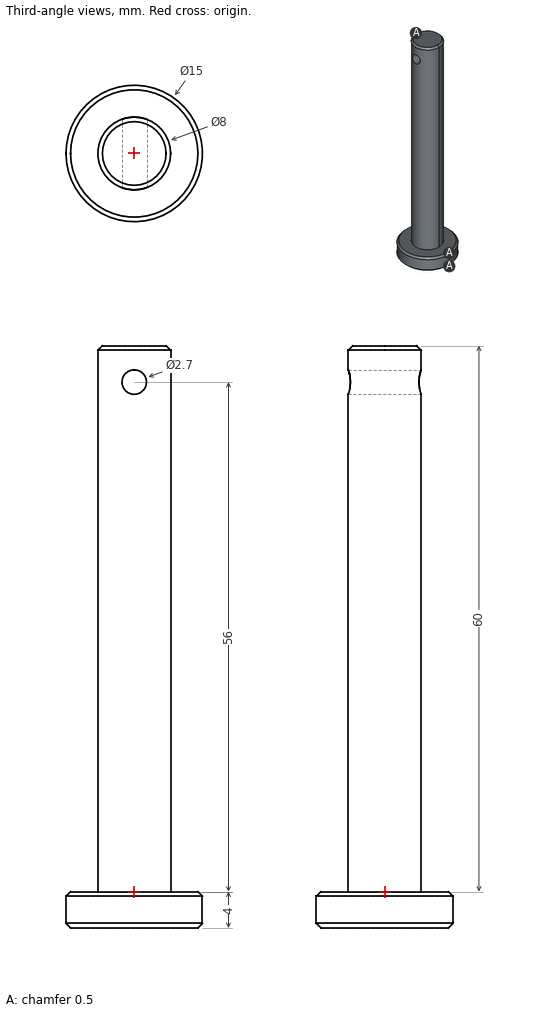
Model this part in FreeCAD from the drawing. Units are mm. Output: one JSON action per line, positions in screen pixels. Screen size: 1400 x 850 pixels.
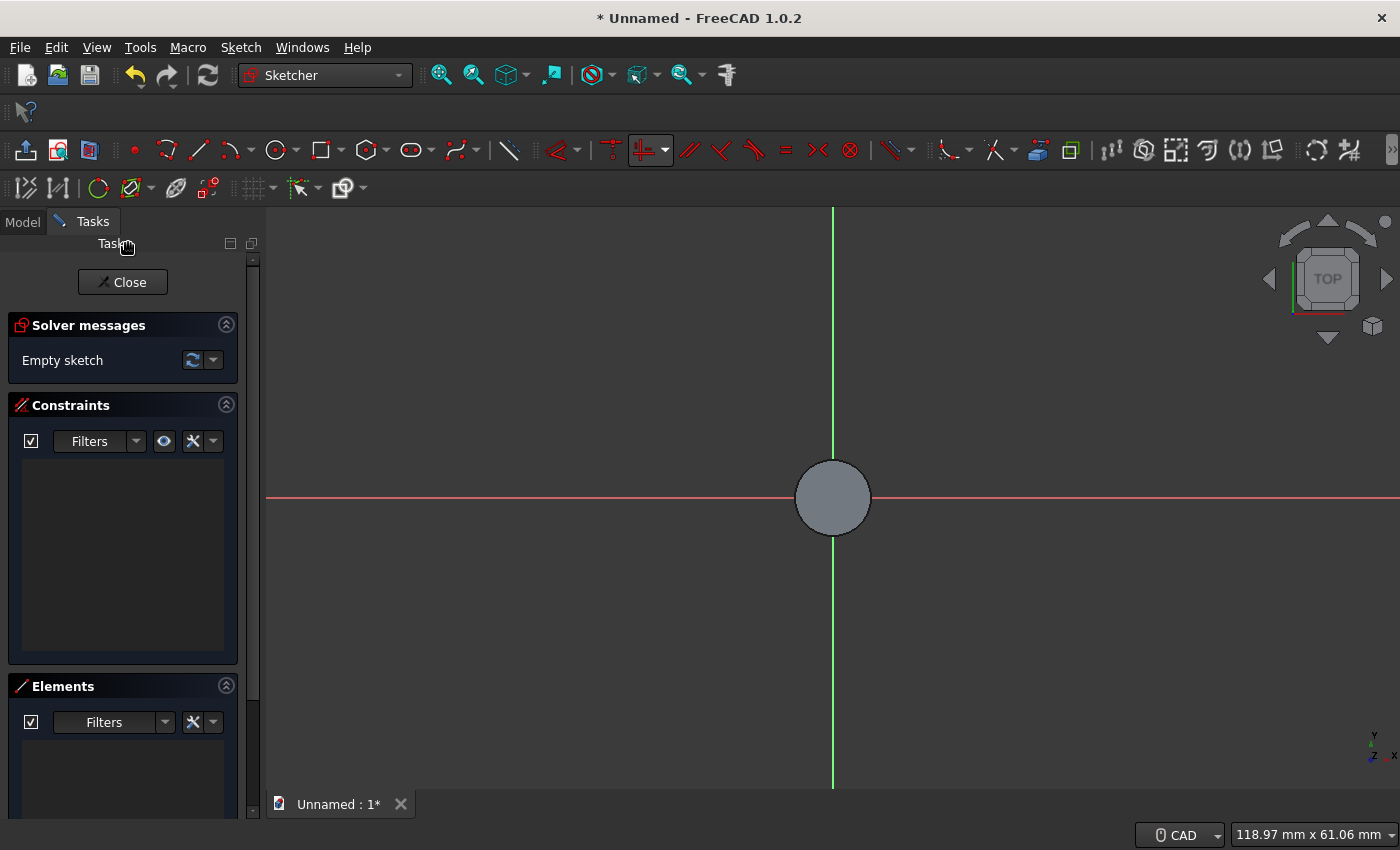
{"action": "left_click", "coordinate": [90, 150]}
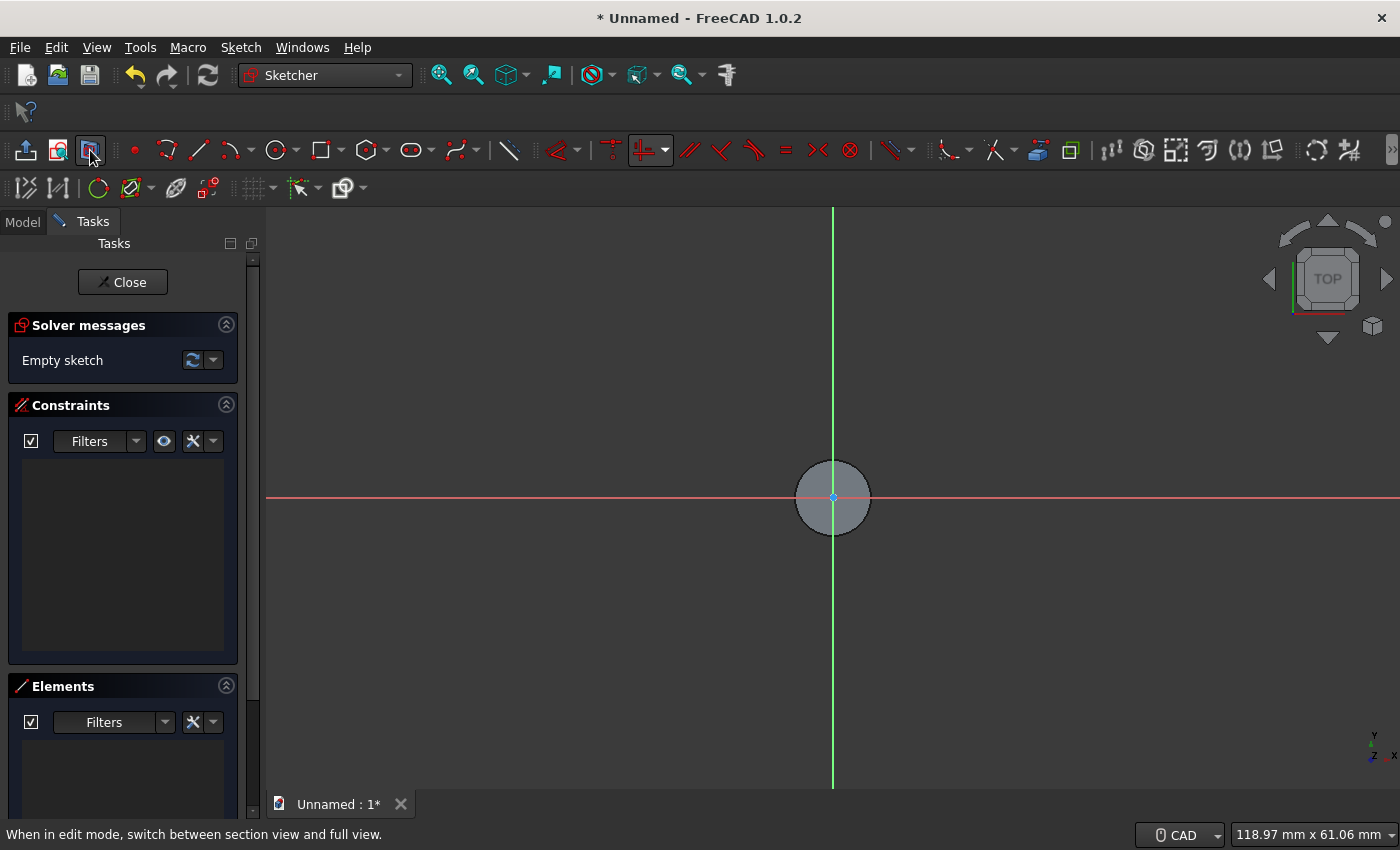
{"action": "scroll", "coordinate": [873, 498], "scroll_direction": "up", "scroll_amount": 5}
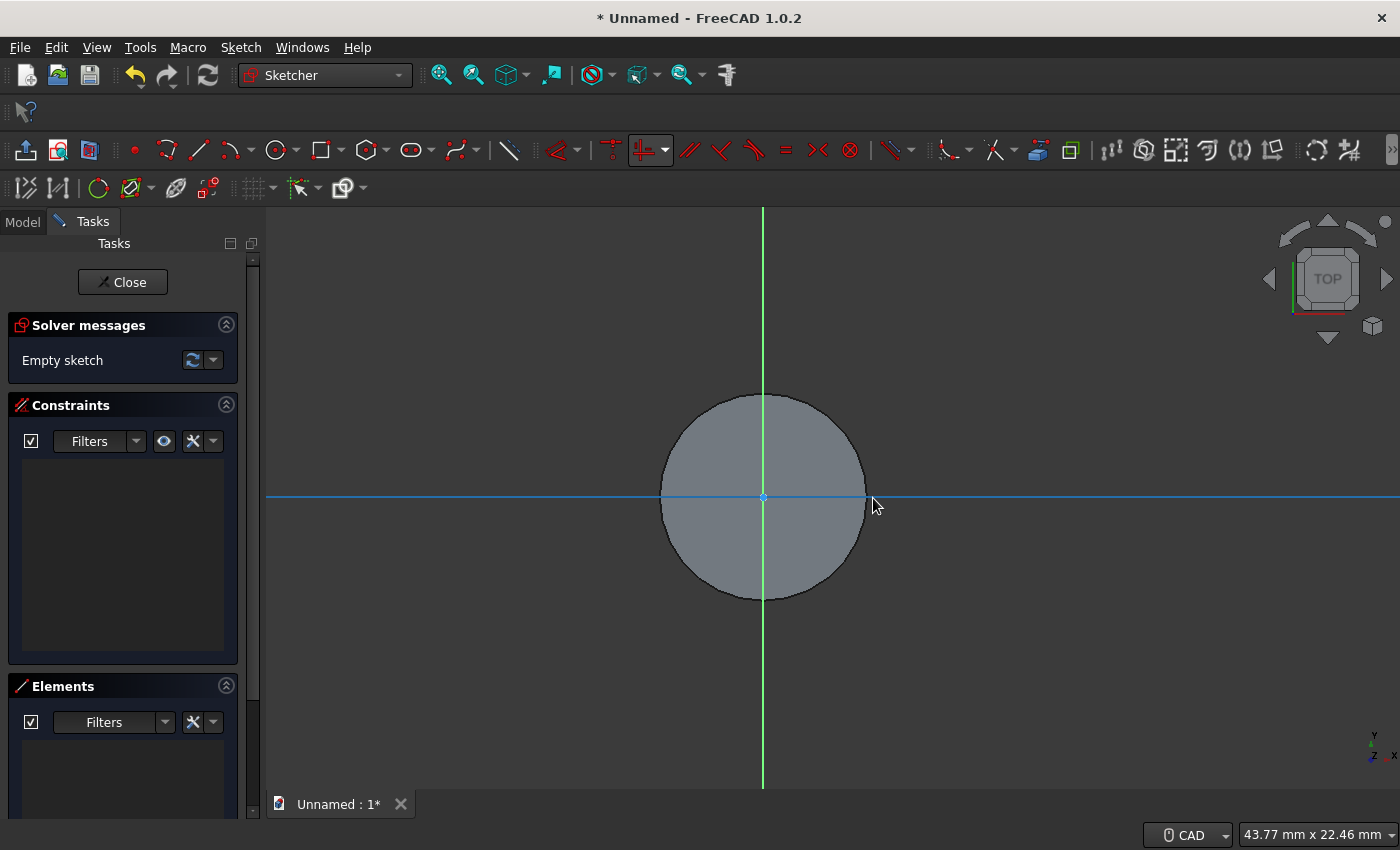
{"action": "left_click", "coordinate": [276, 150]}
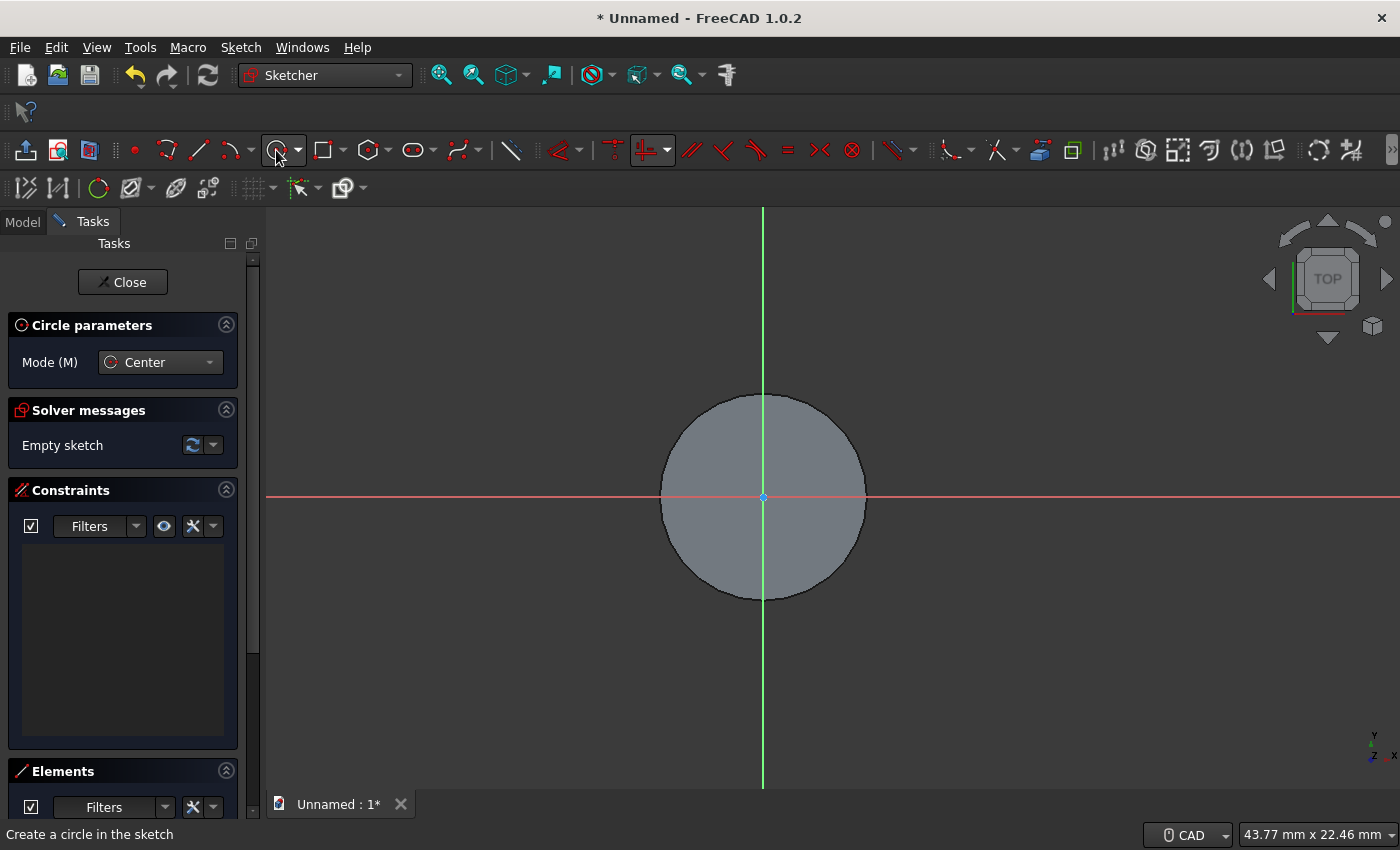
{"action": "left_click", "coordinate": [763, 497]}
{"action": "left_click", "coordinate": [901, 360]}
{"action": "key", "text": "Escape"}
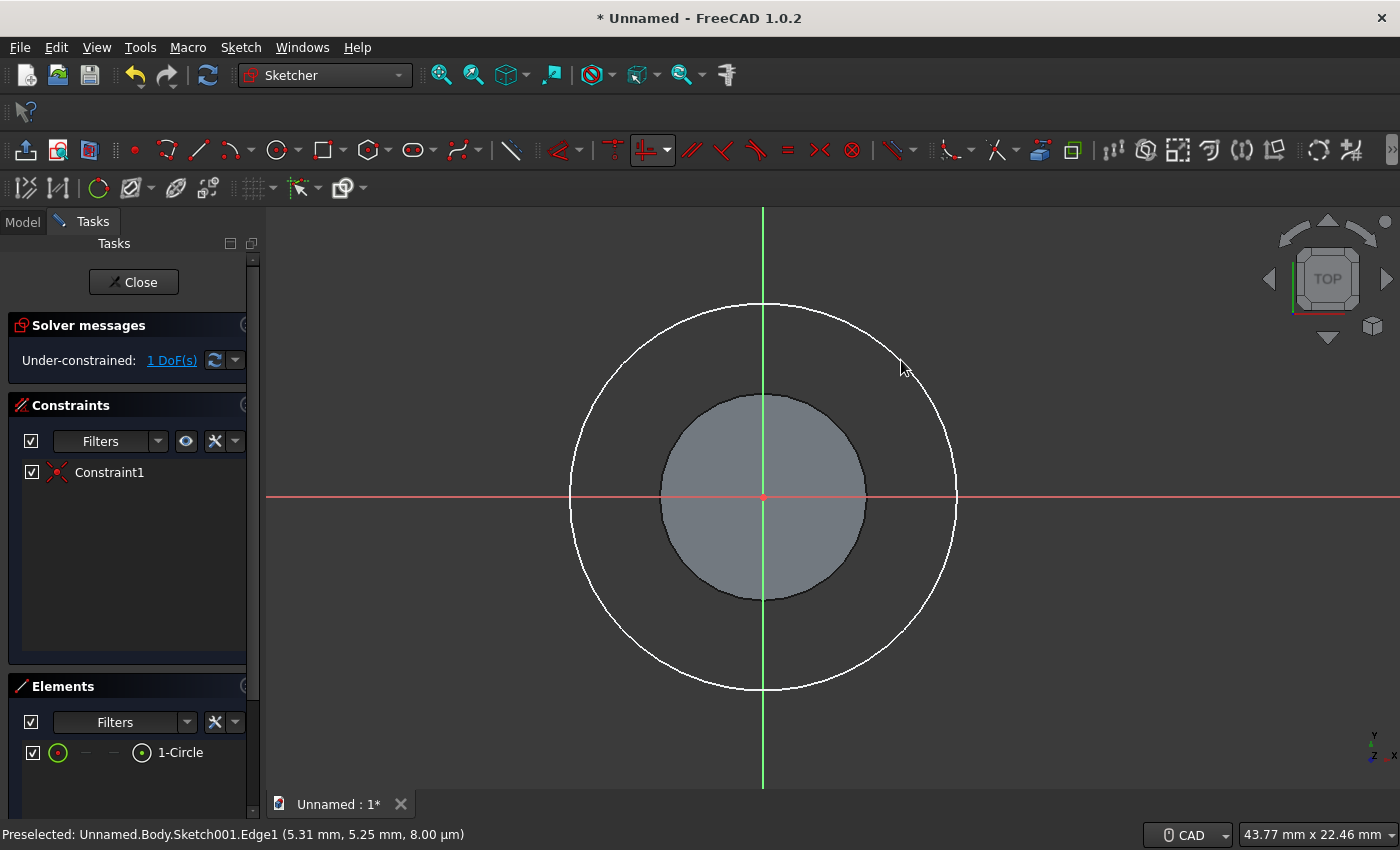
{"action": "left_click", "coordinate": [558, 150]}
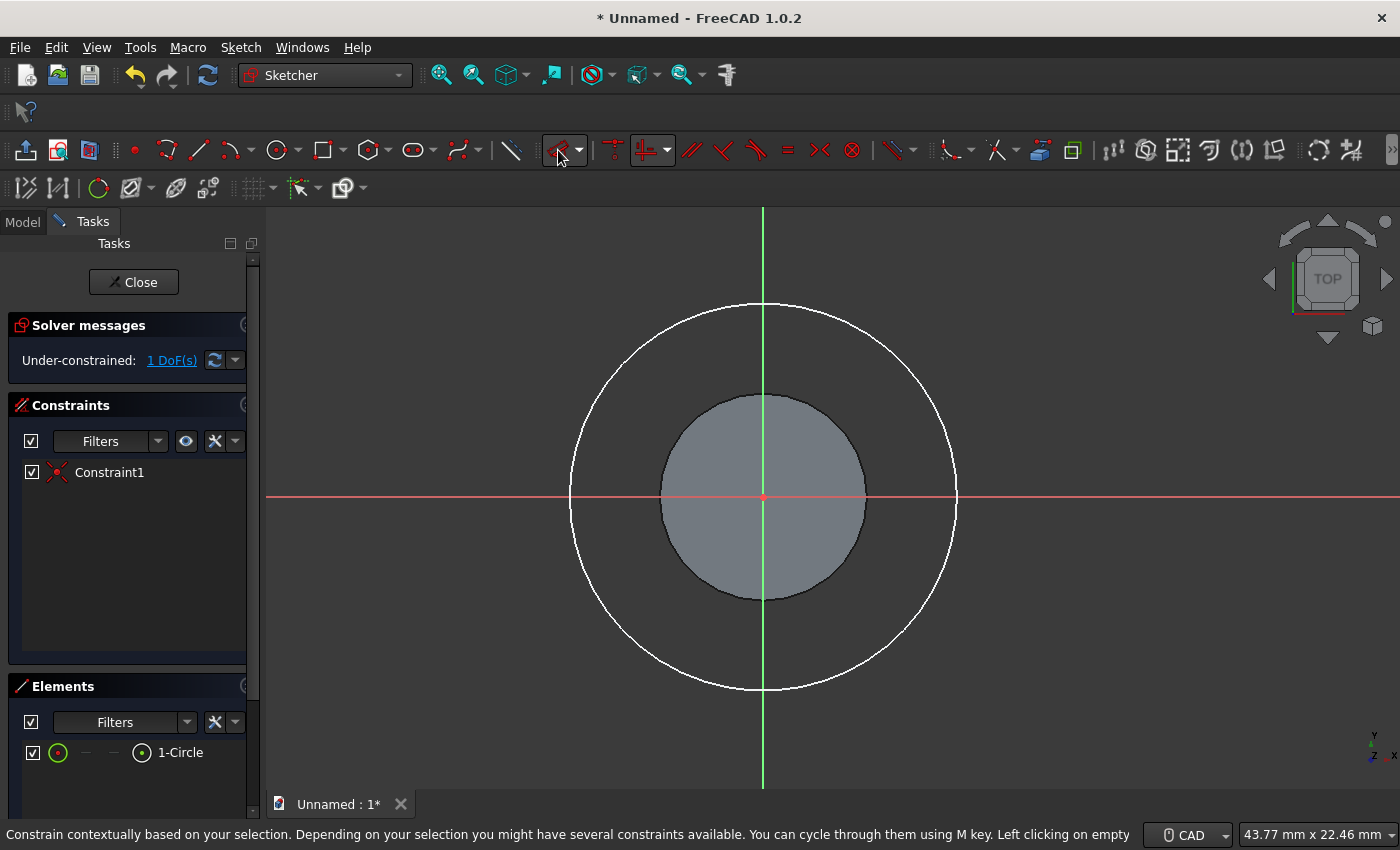
{"action": "left_click", "coordinate": [900, 360]}
{"action": "left_click", "coordinate": [923, 337]}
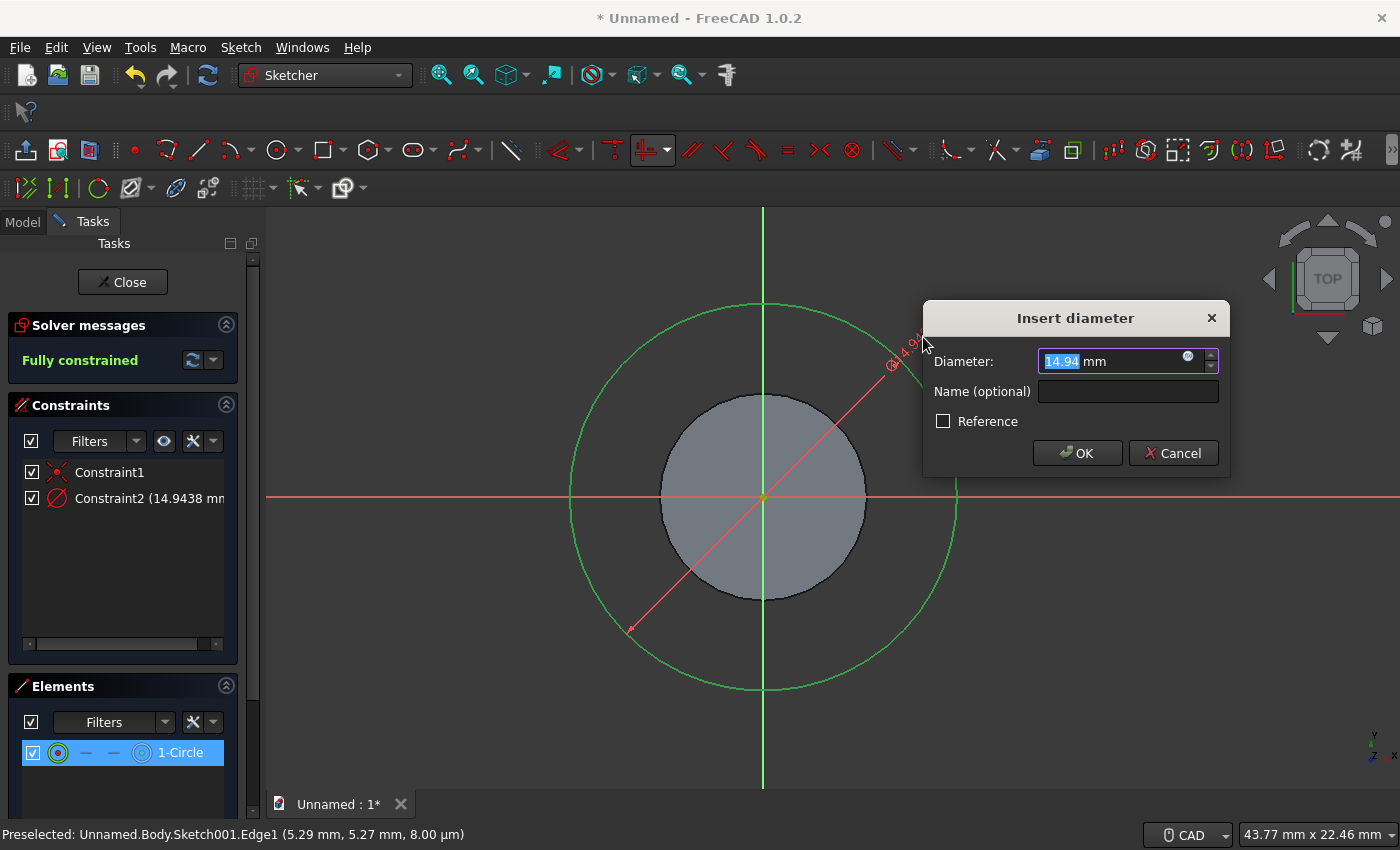
{"action": "type", "text": "15"}
{"action": "key", "text": "Return"}
{"action": "key", "text": "Escape"}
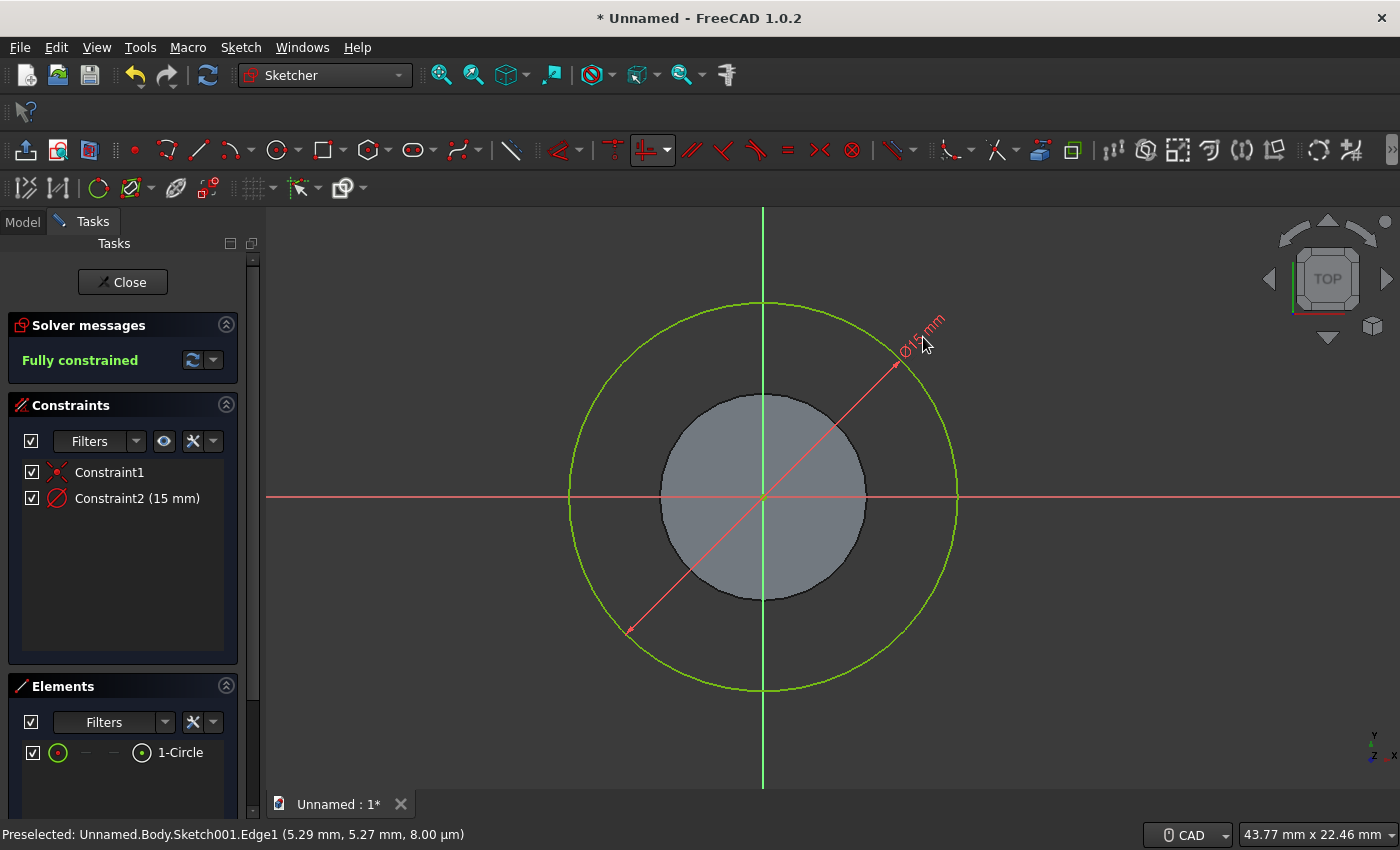
{"action": "left_click", "coordinate": [123, 282]}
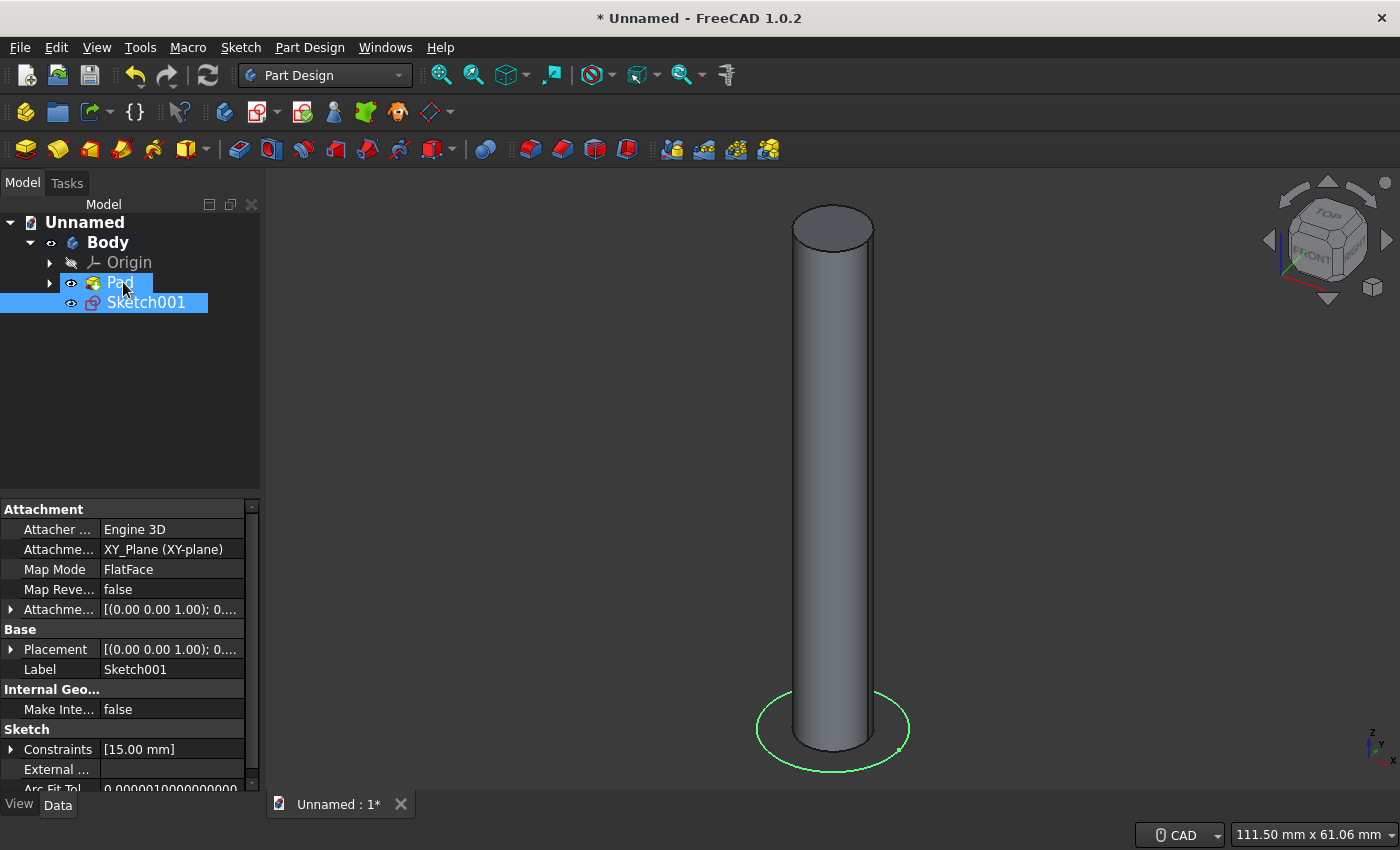
{"action": "left_click", "coordinate": [26, 150]}